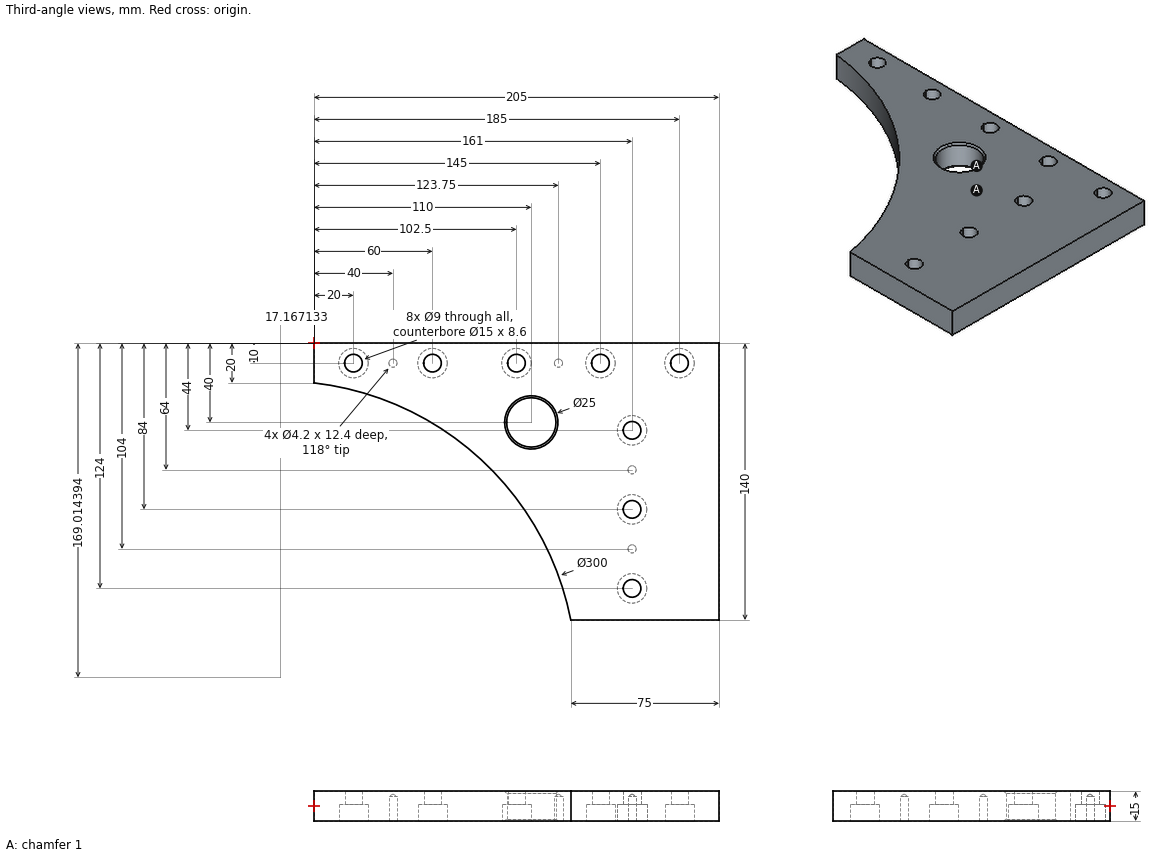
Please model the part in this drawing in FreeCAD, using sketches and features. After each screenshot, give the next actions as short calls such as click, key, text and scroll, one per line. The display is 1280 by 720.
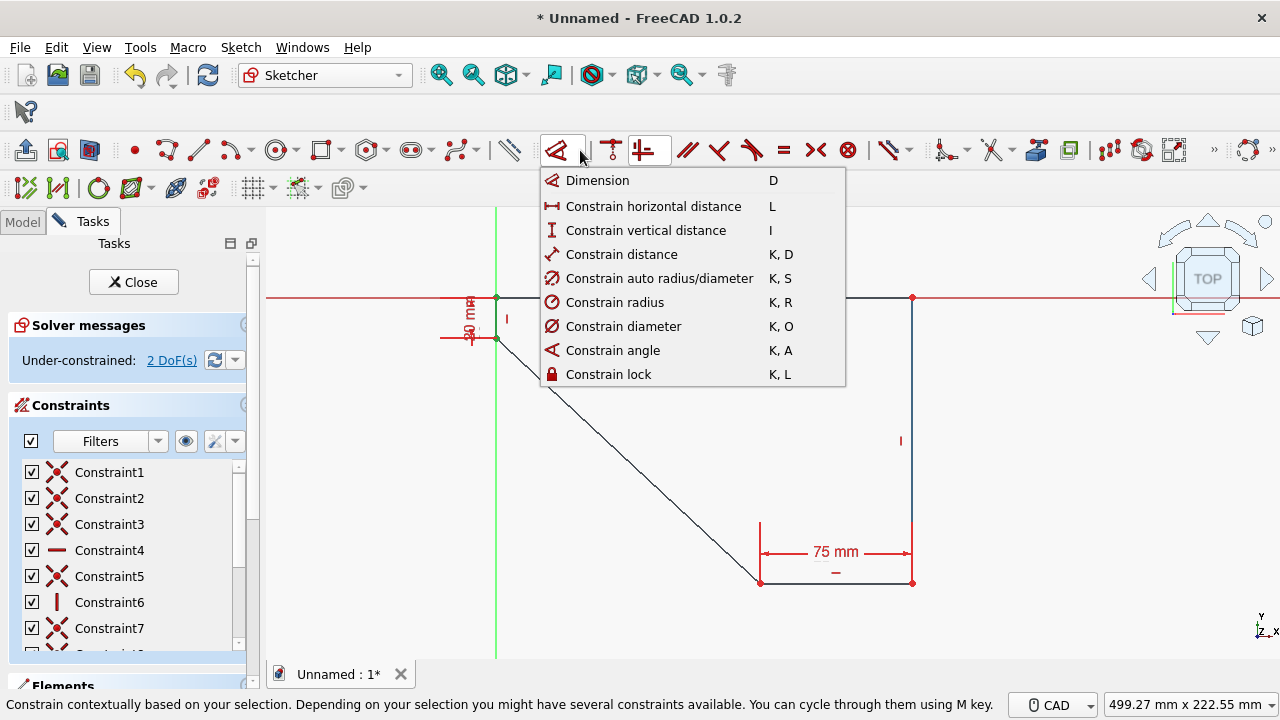
click(693, 230)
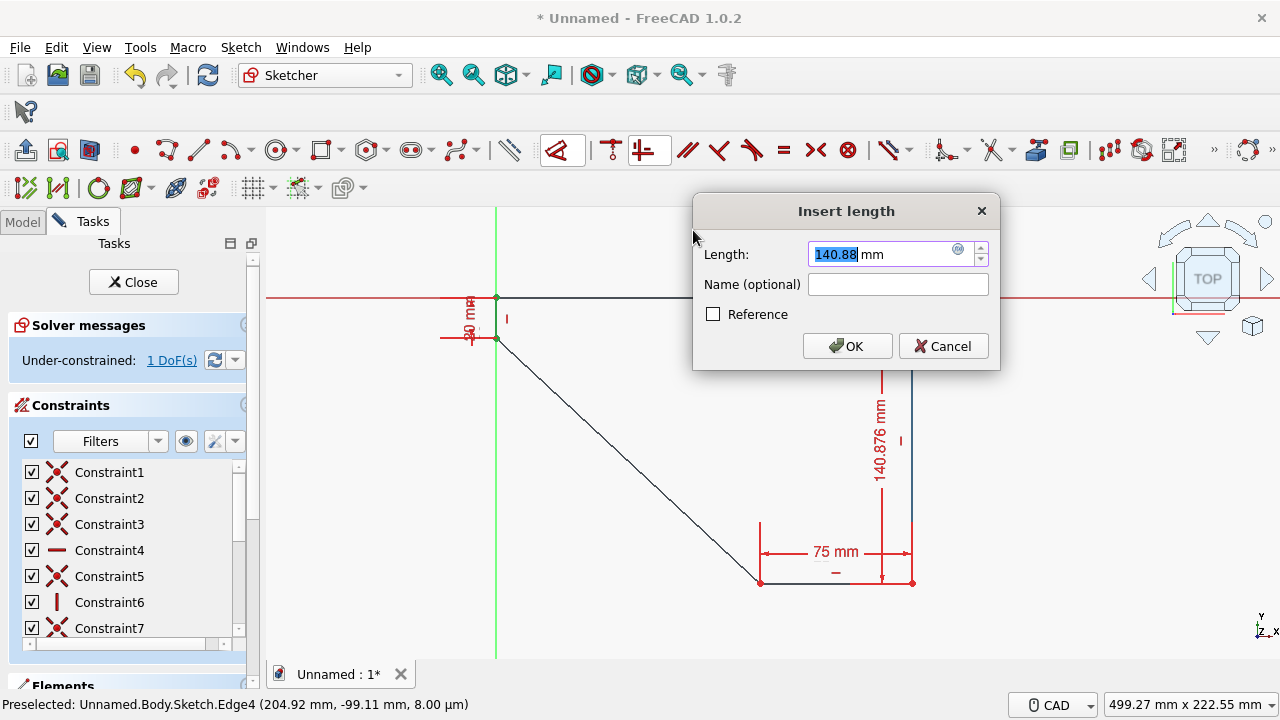
text(140)
key(Return)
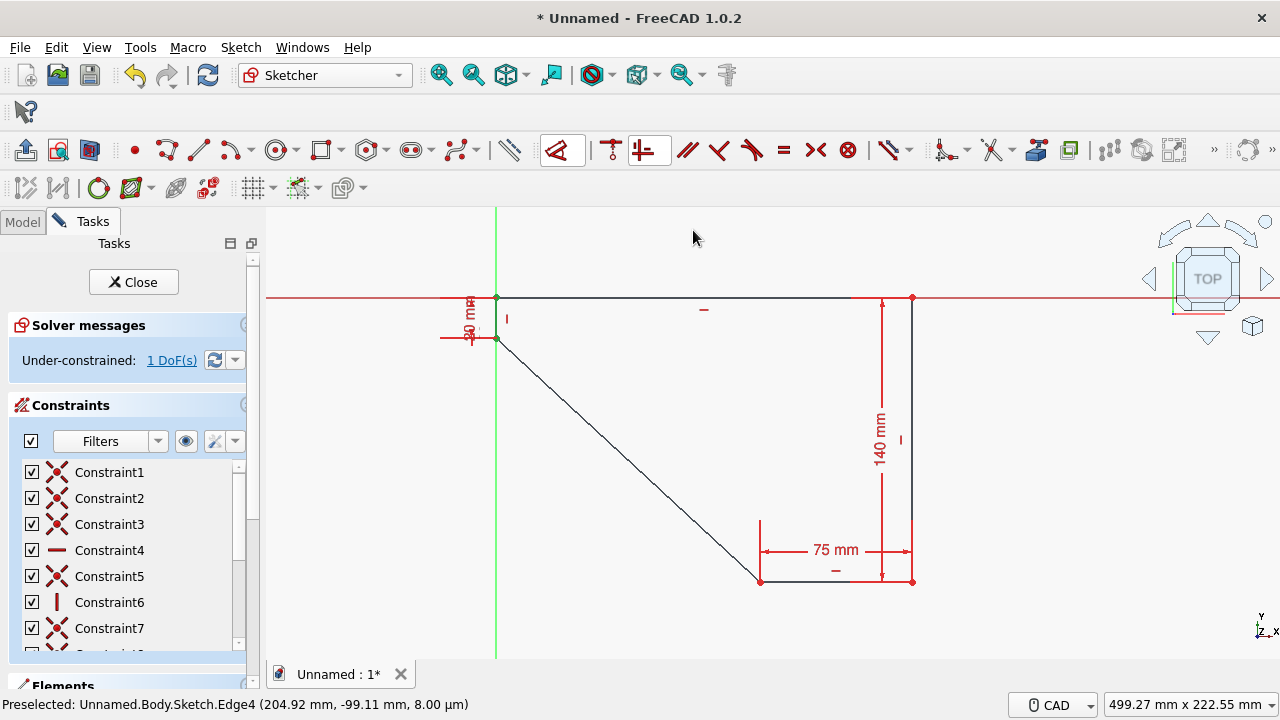
click(788, 298)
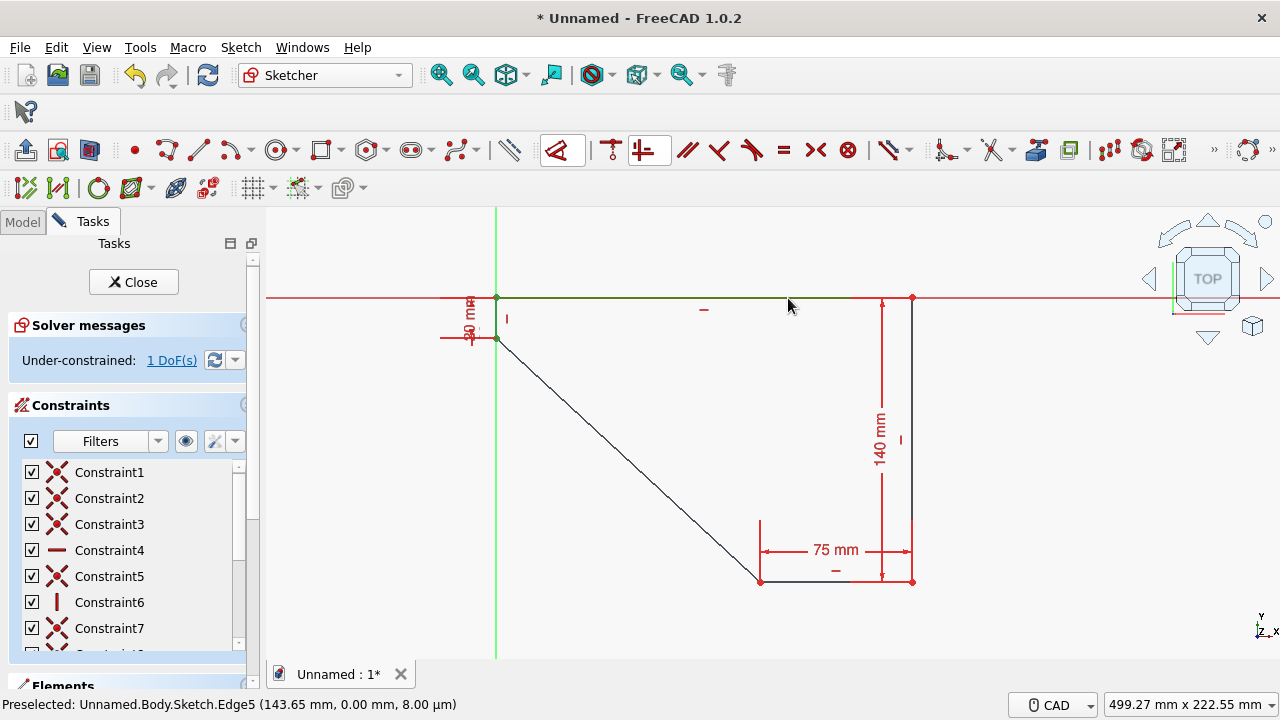
key(l)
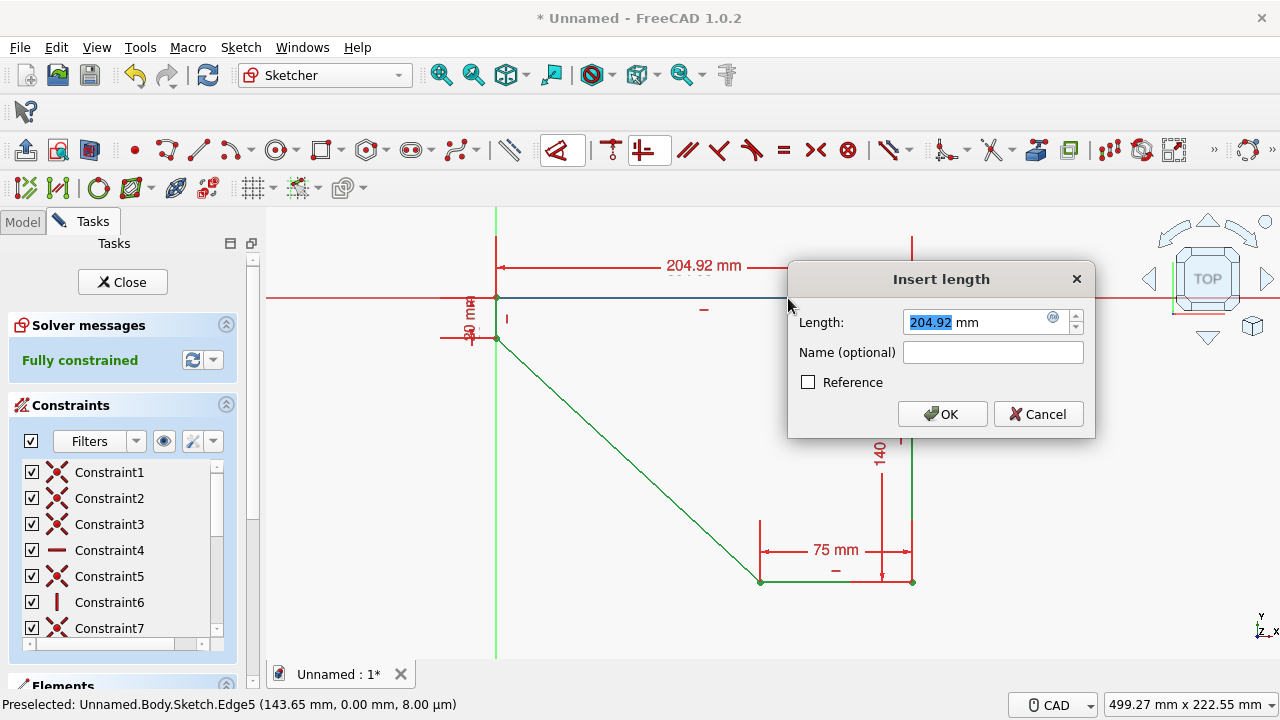
text(205)
key(Return)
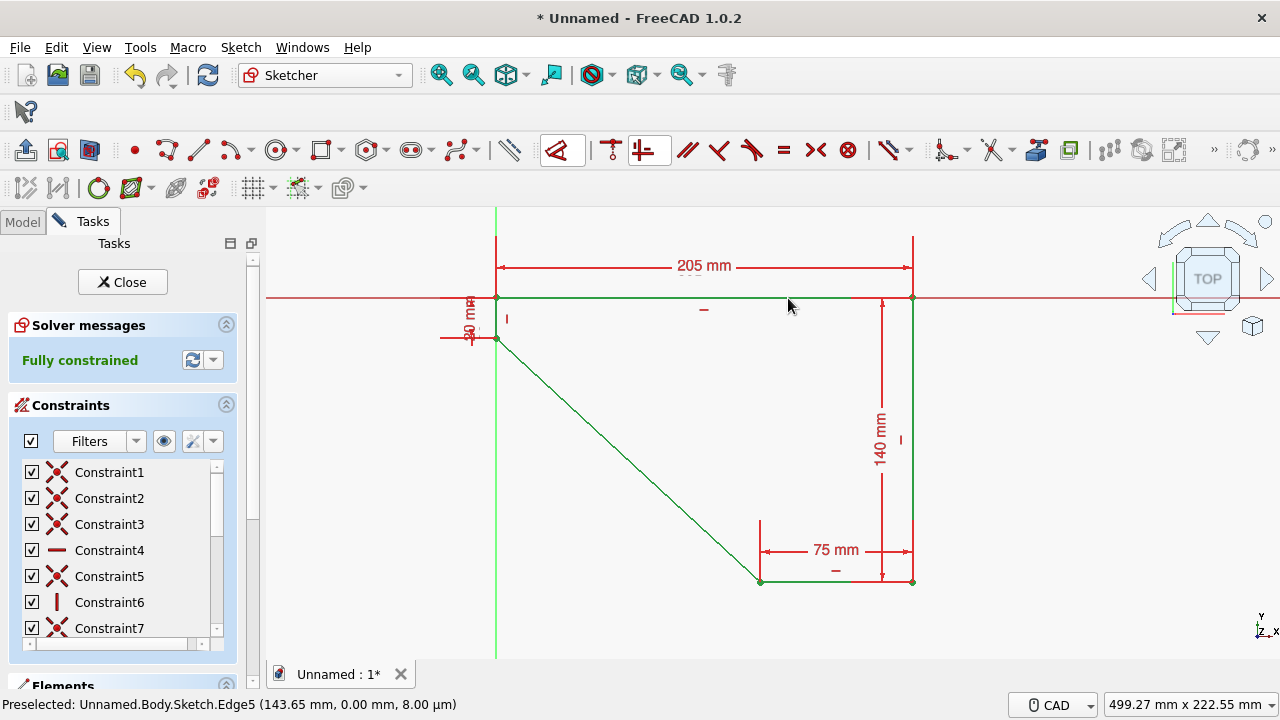
click(123, 282)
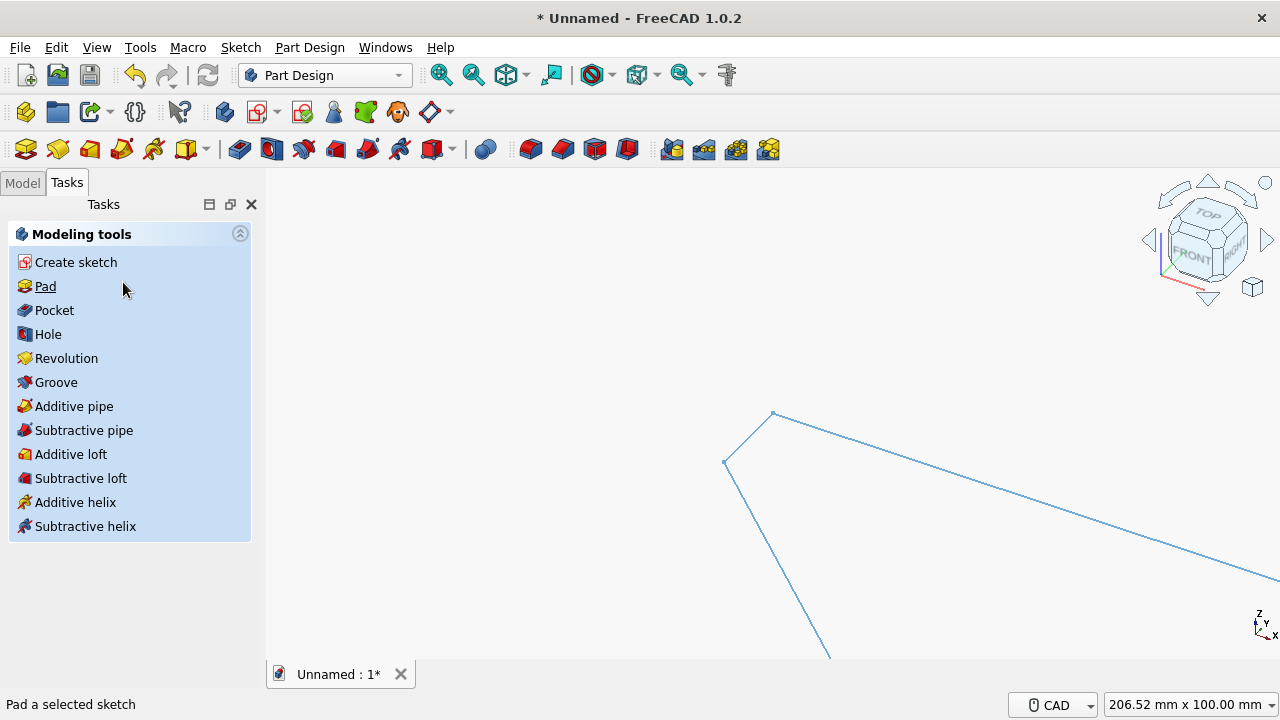
click(26, 150)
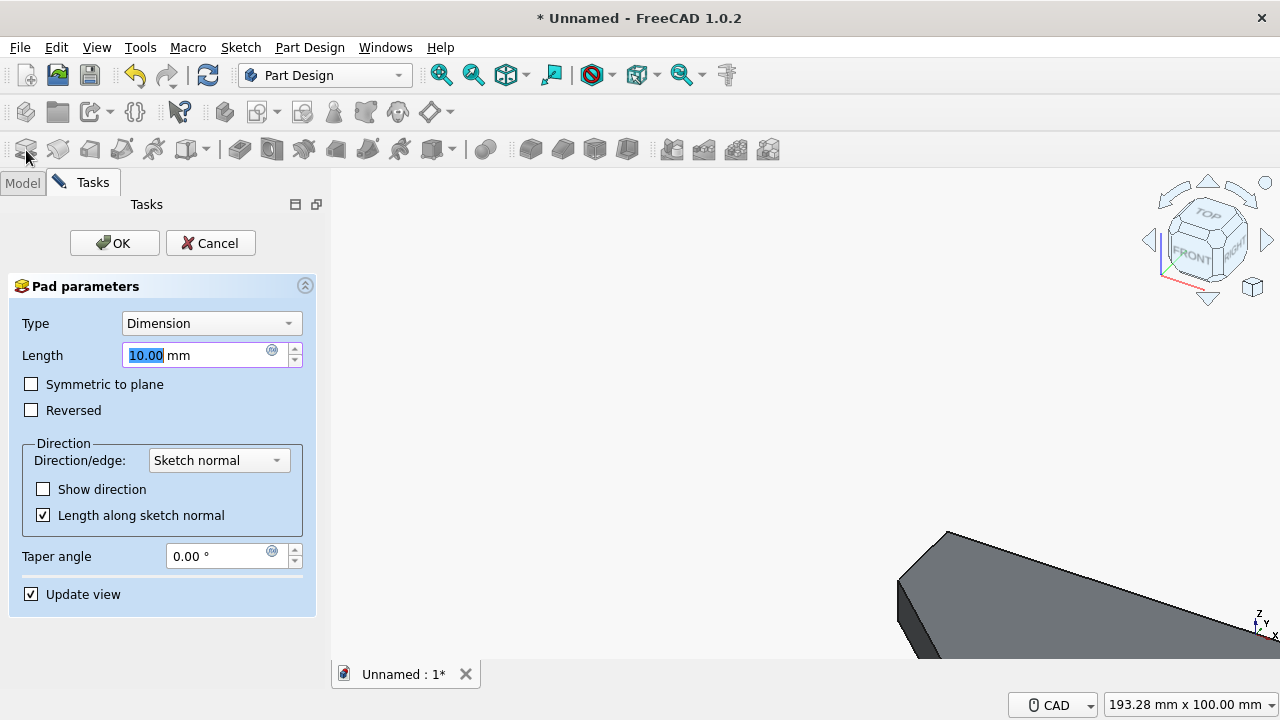
text(15)
key(Tab)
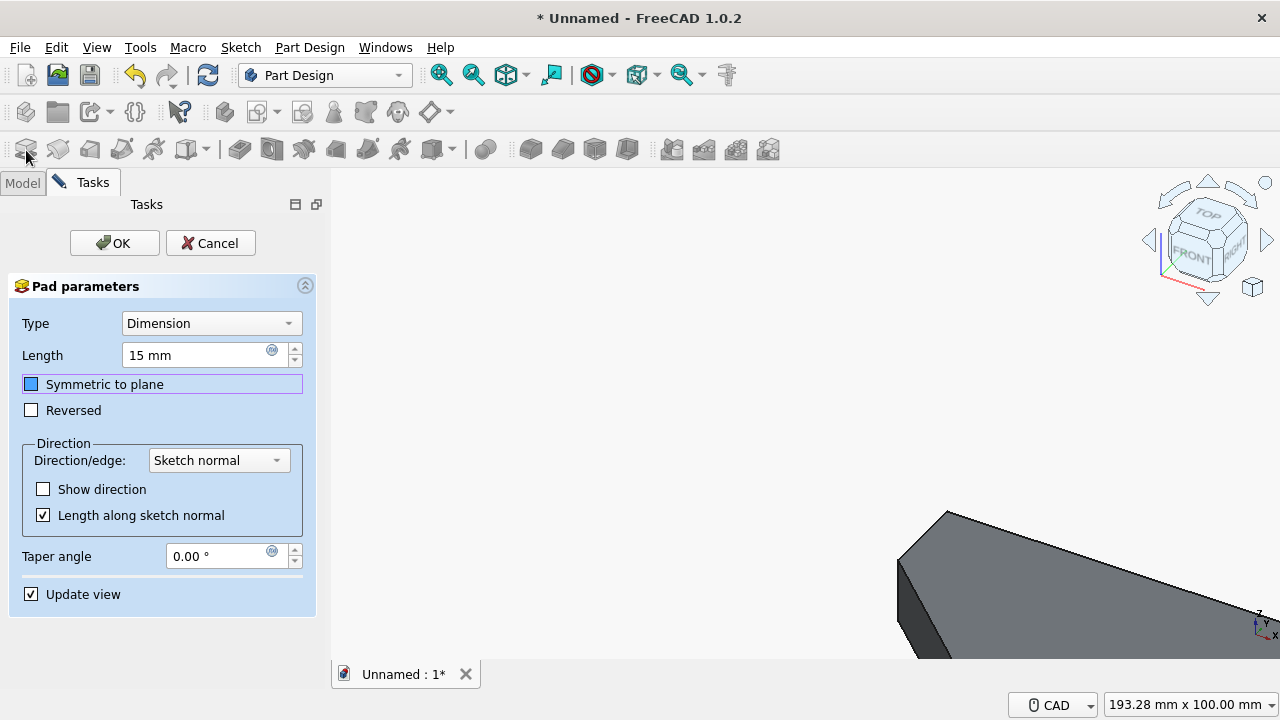
click(30, 384)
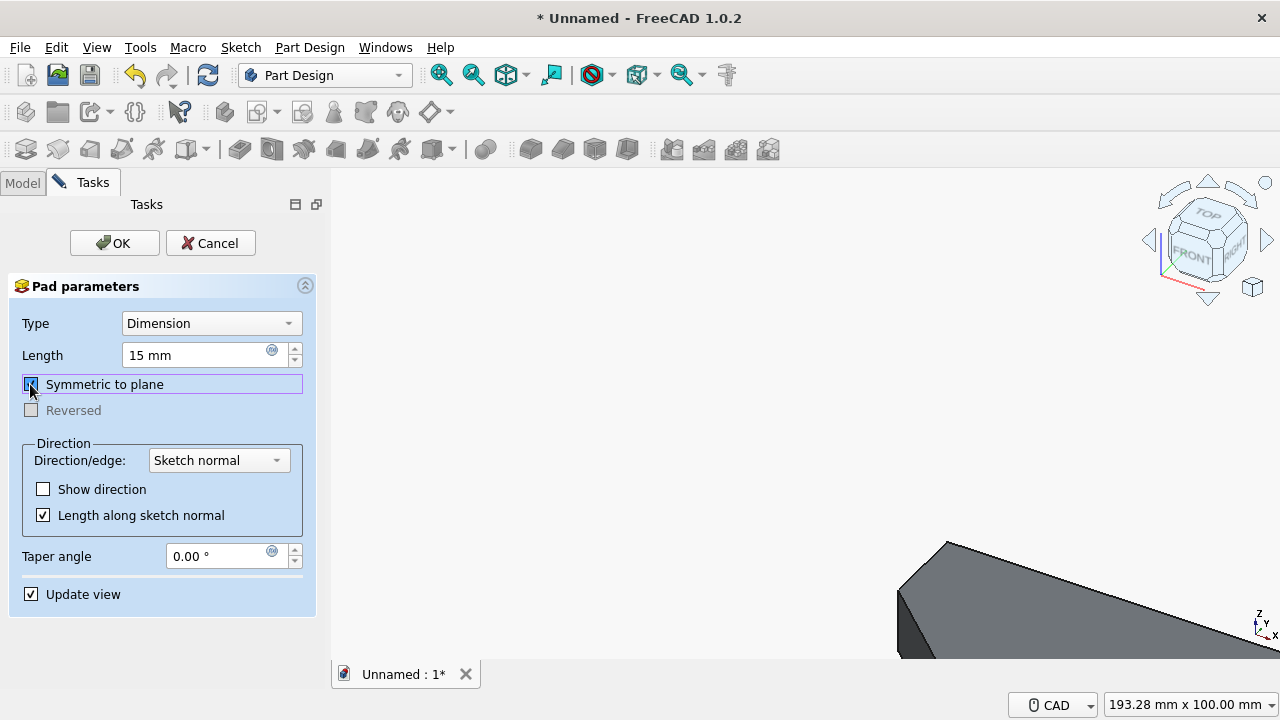
click(115, 243)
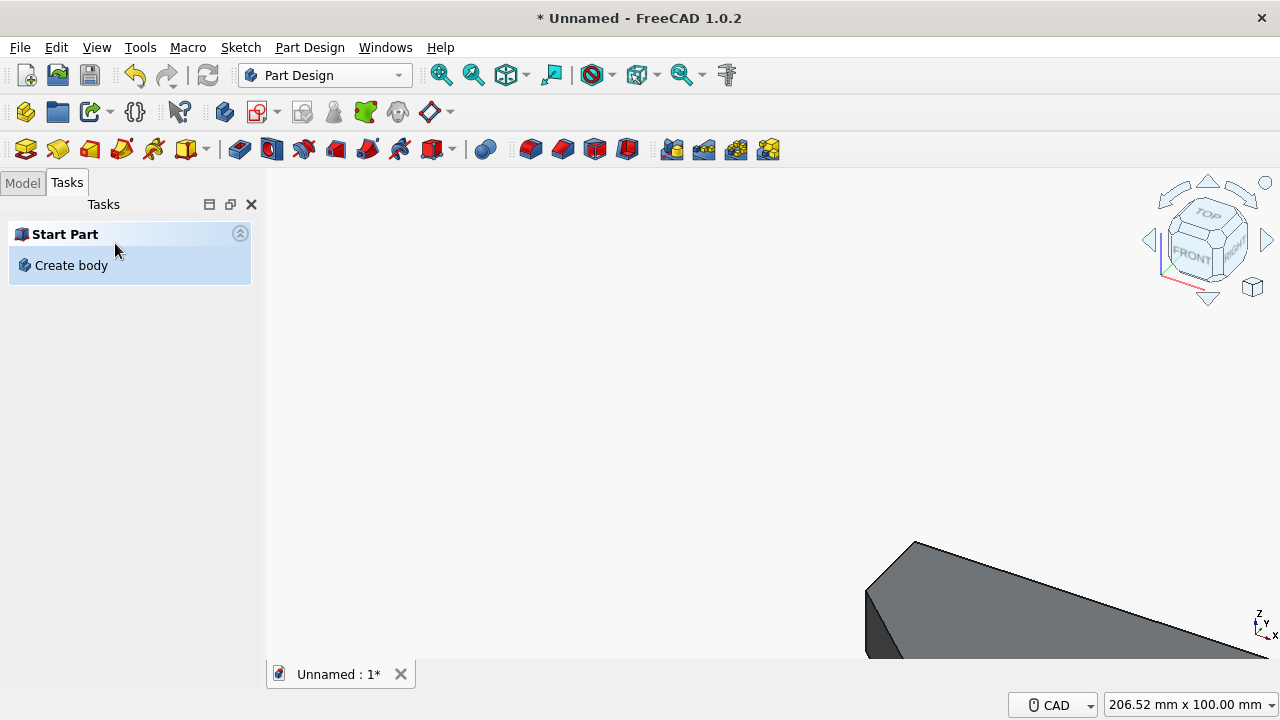
click(442, 76)